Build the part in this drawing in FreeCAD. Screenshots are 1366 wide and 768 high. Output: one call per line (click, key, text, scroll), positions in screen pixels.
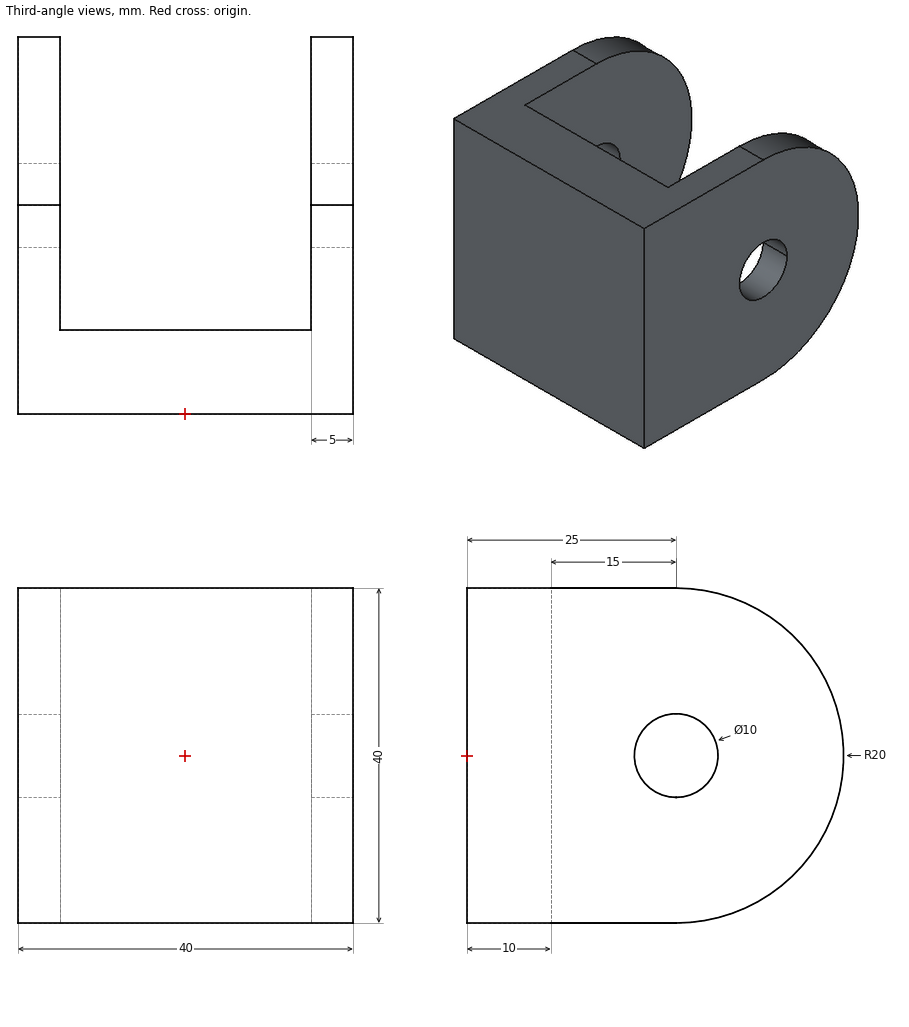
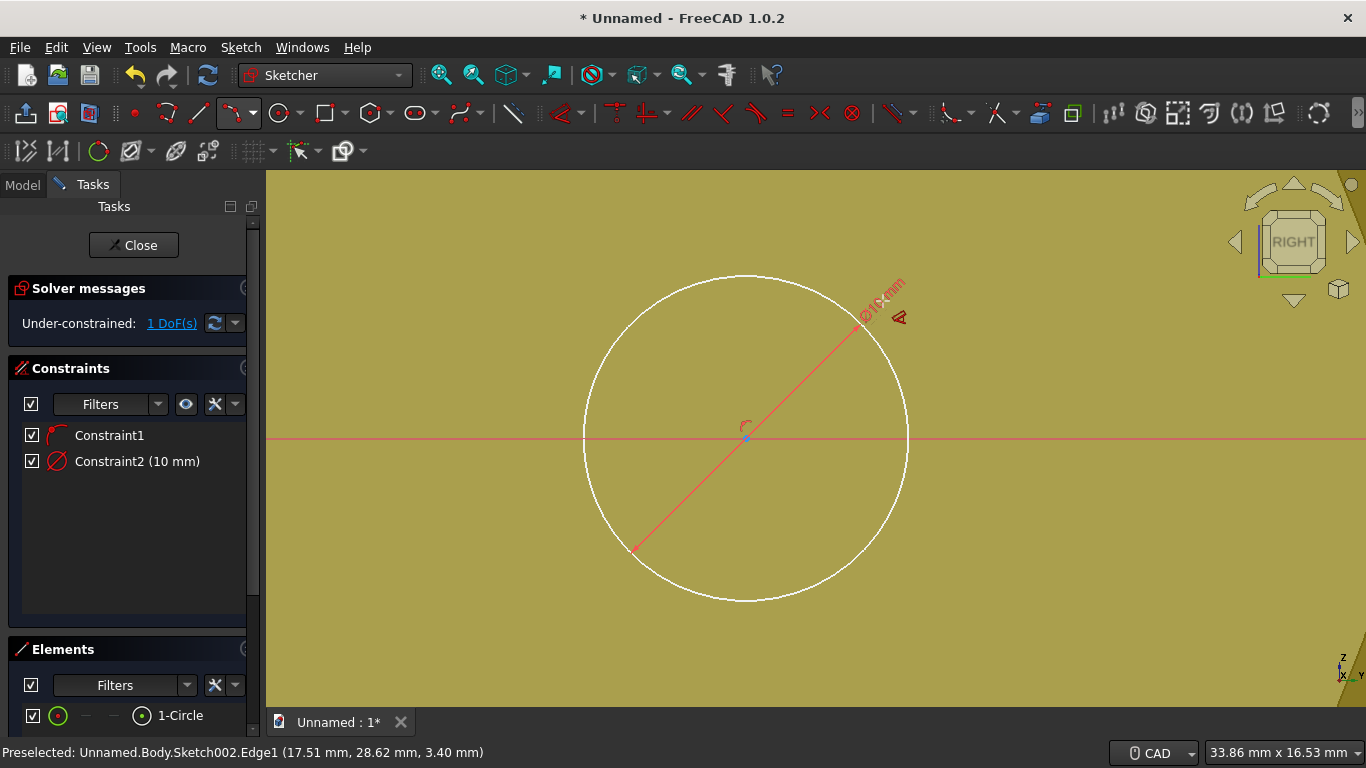
click(746, 438)
click(520, 472)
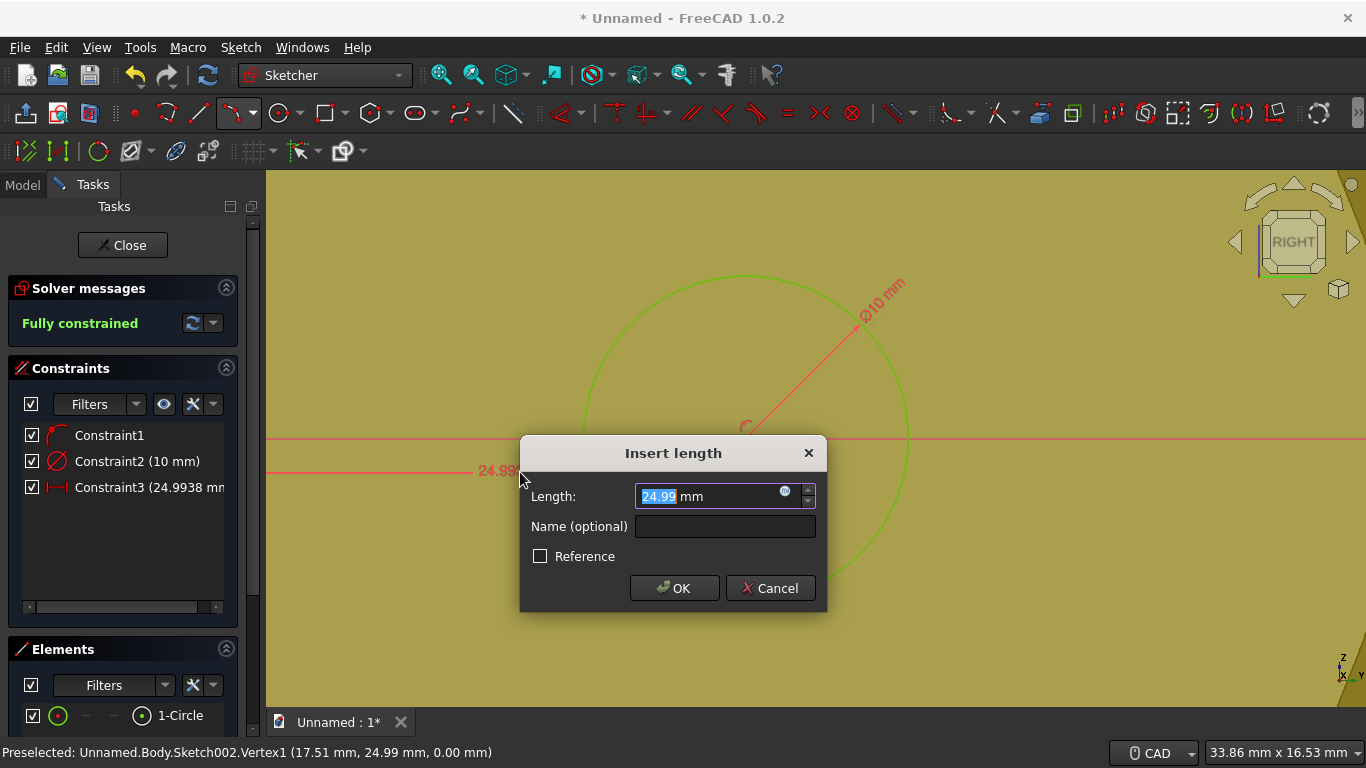
text(25)
key(Return)
key(Escape)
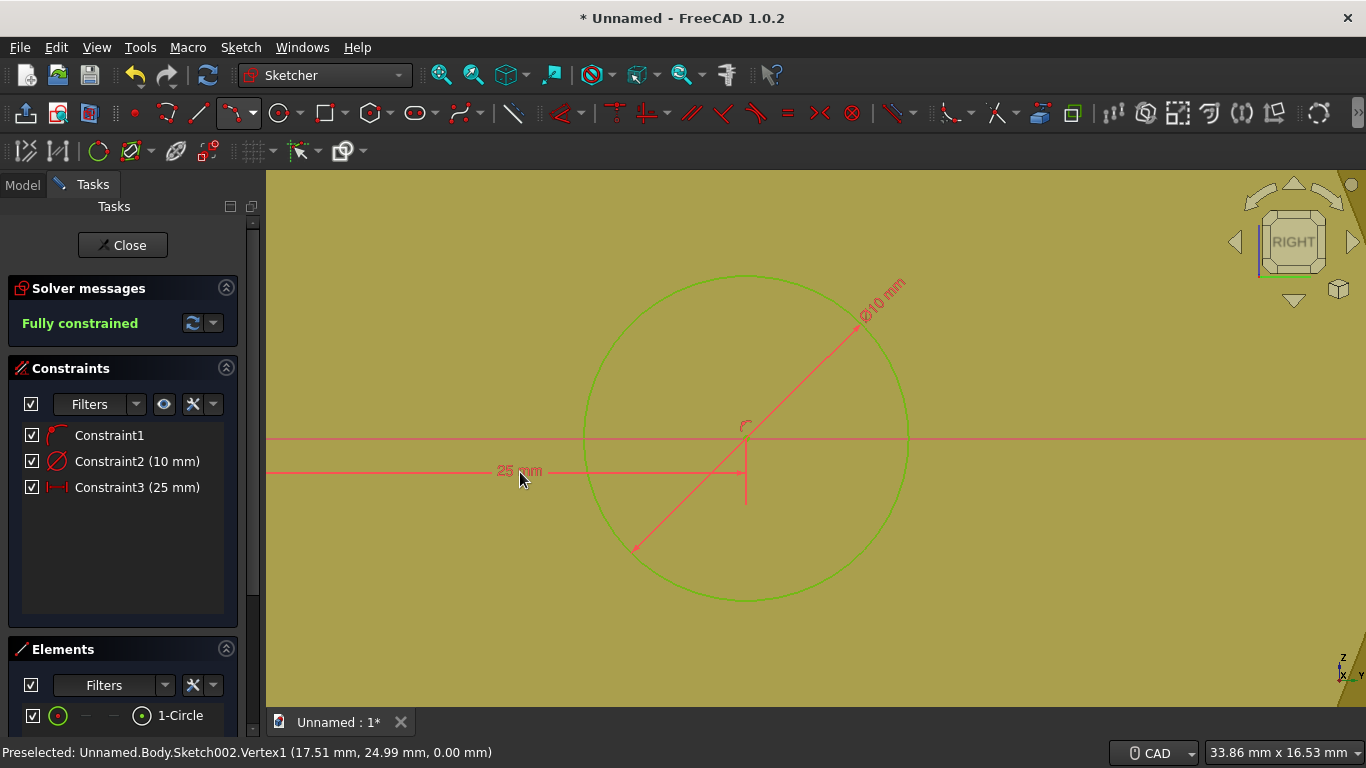
click(123, 245)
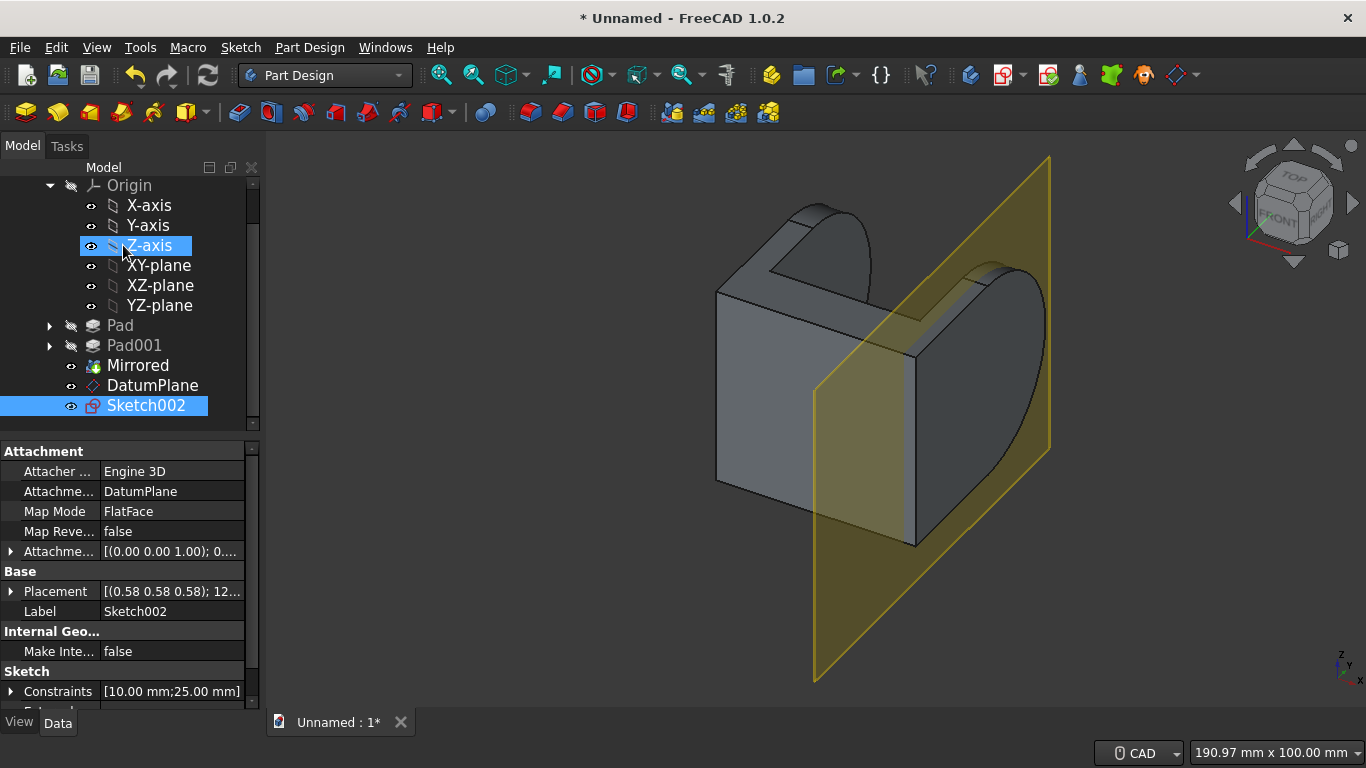
click(240, 112)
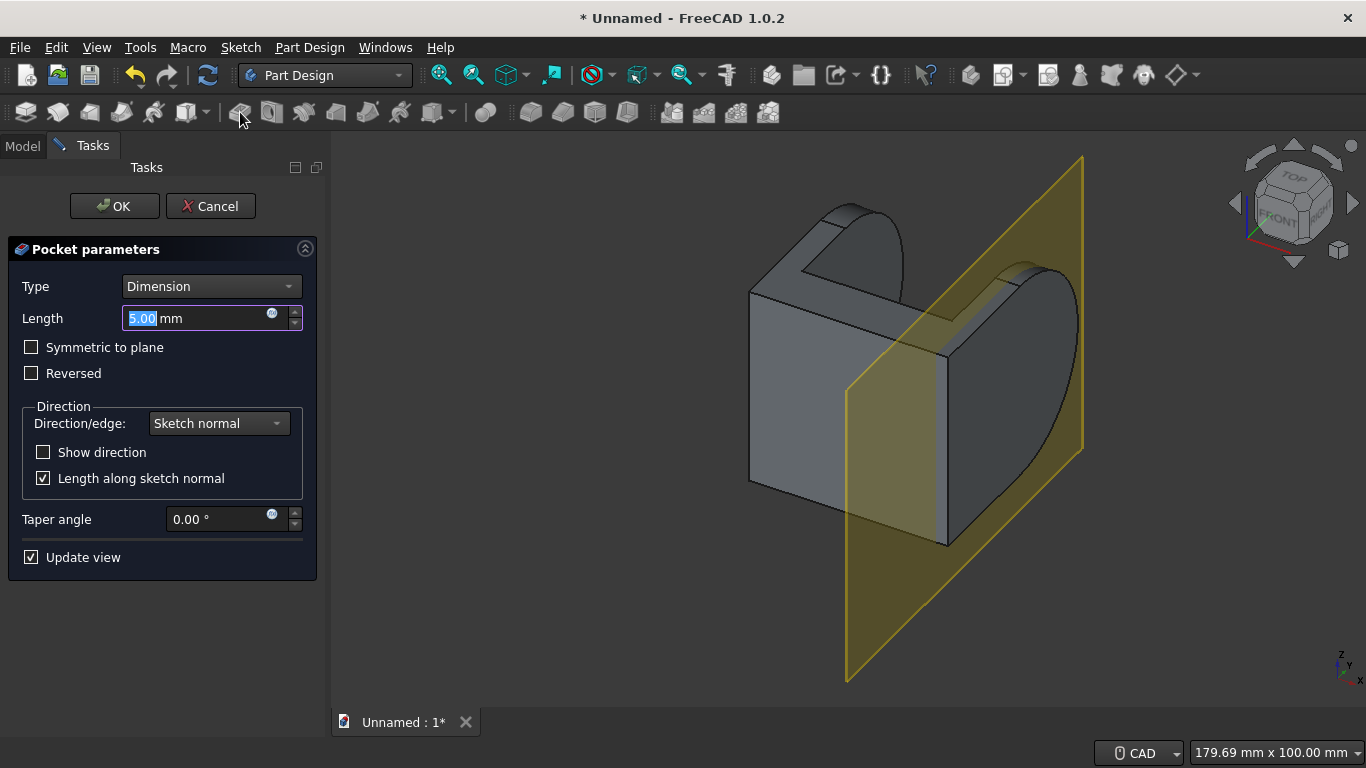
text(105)
key(Tab)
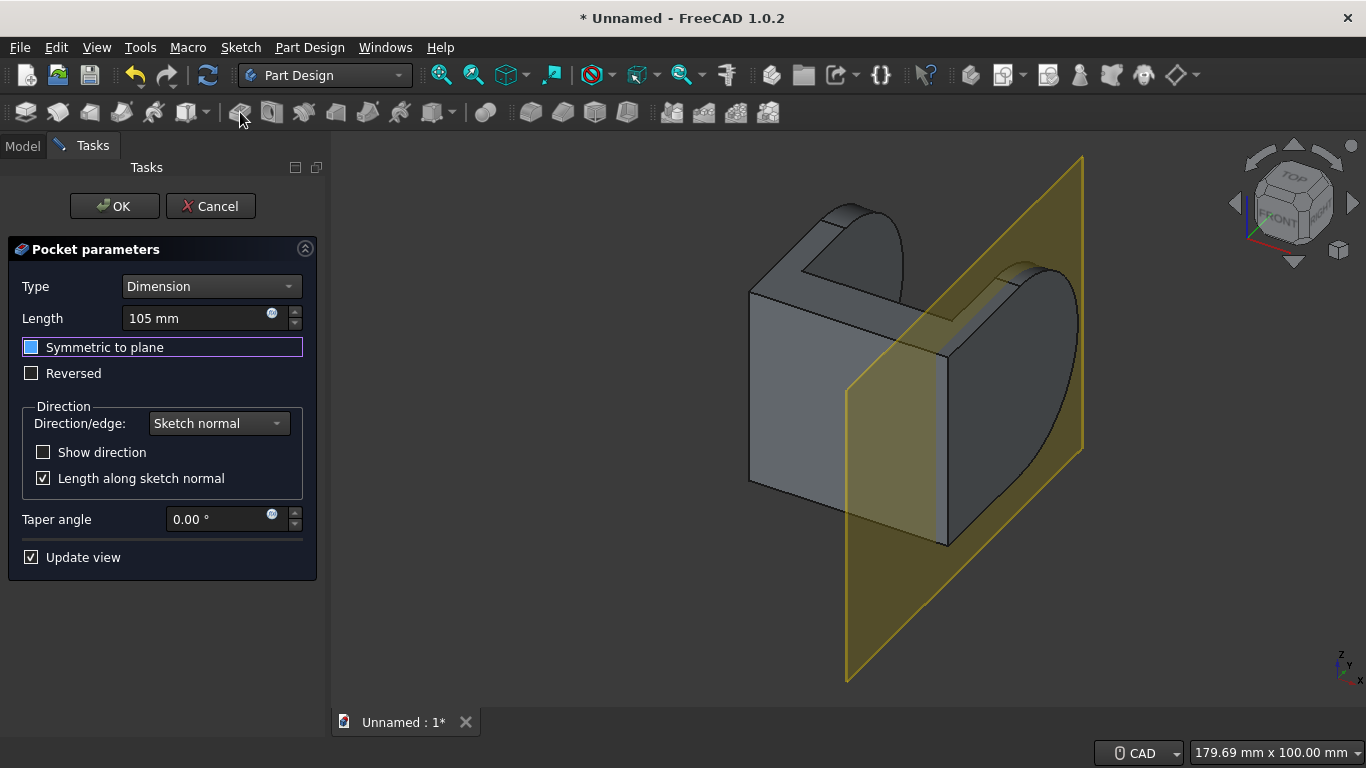
click(30, 347)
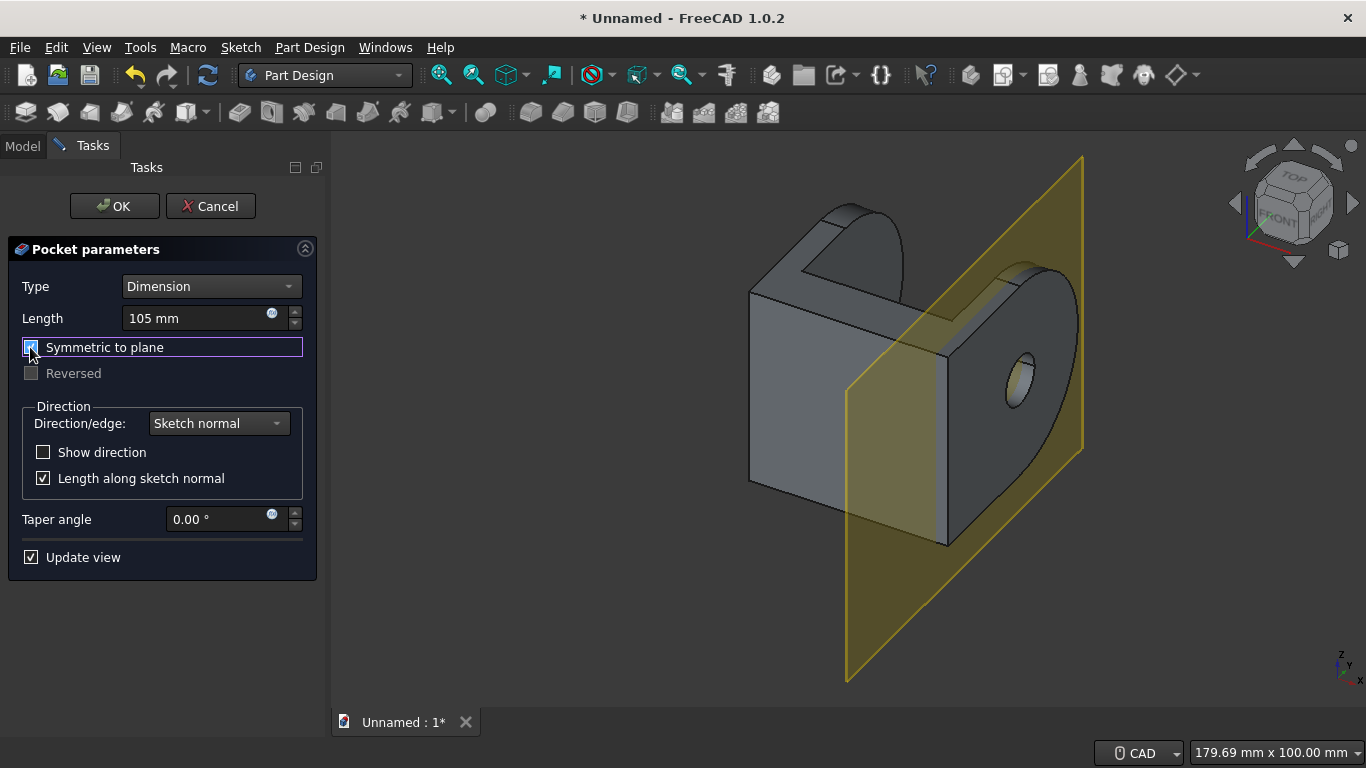
click(115, 206)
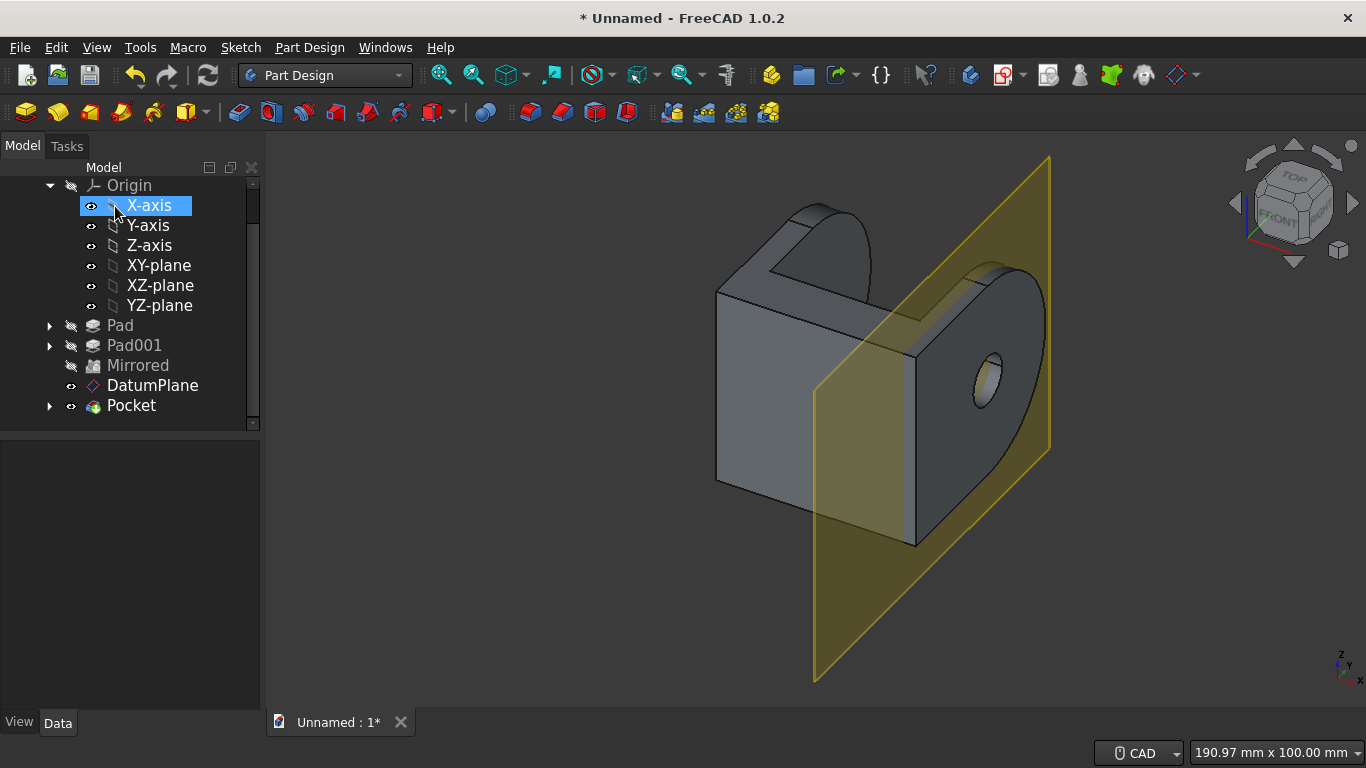
click(116, 386)
key(space)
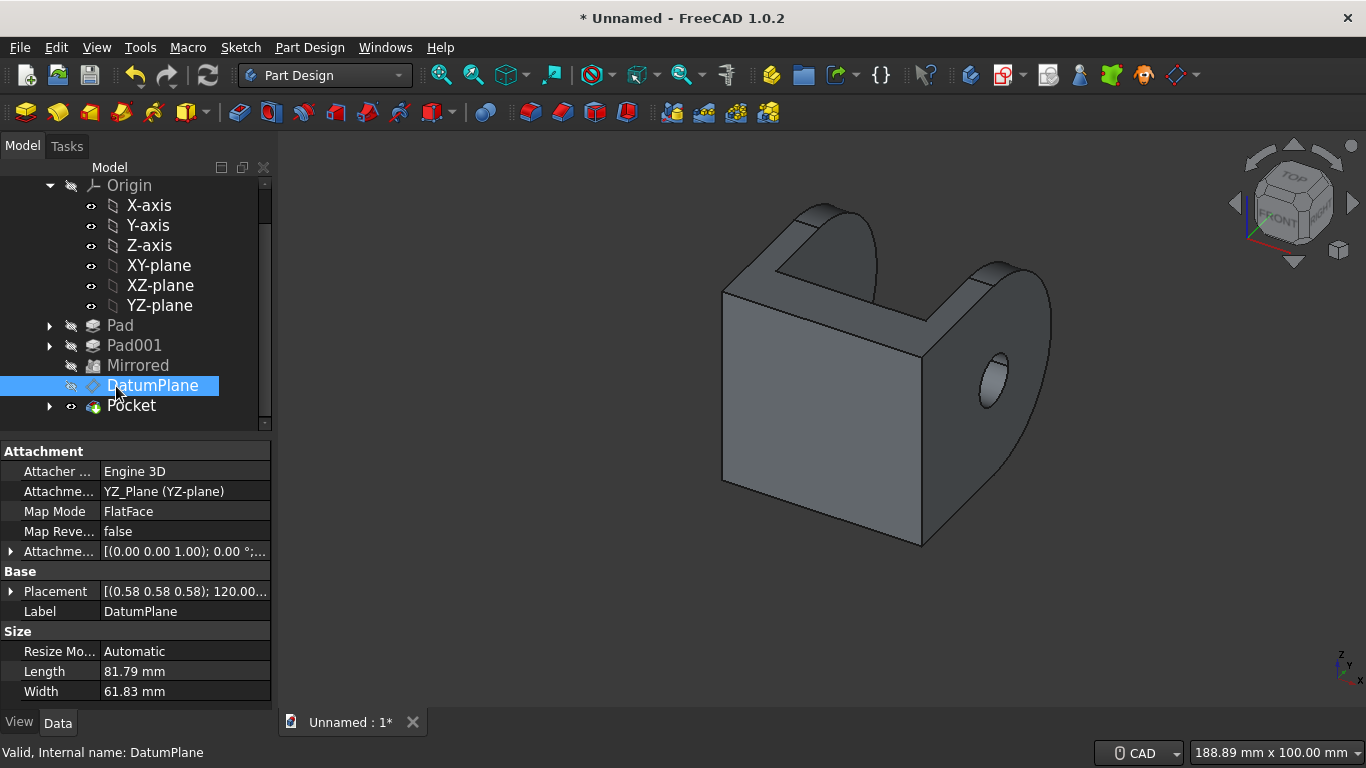
key(0)